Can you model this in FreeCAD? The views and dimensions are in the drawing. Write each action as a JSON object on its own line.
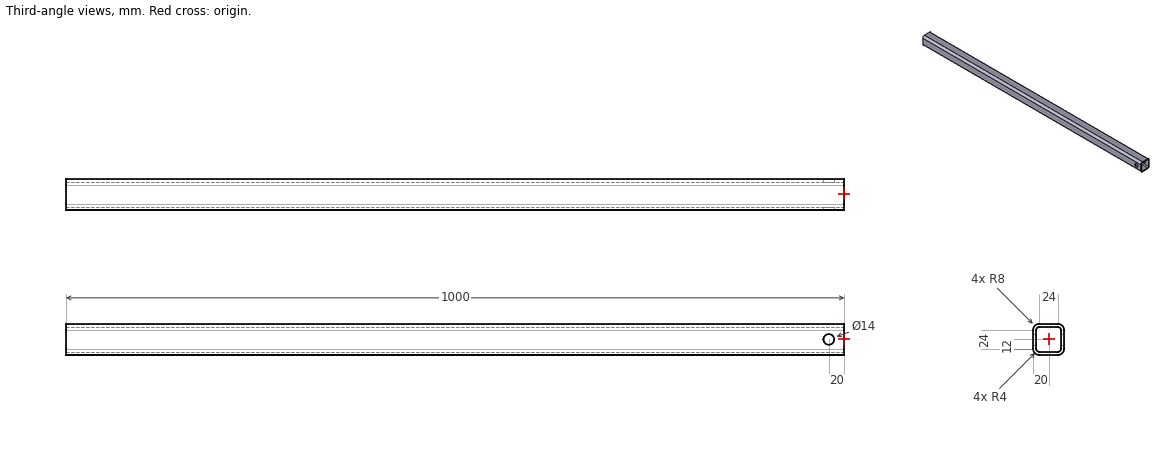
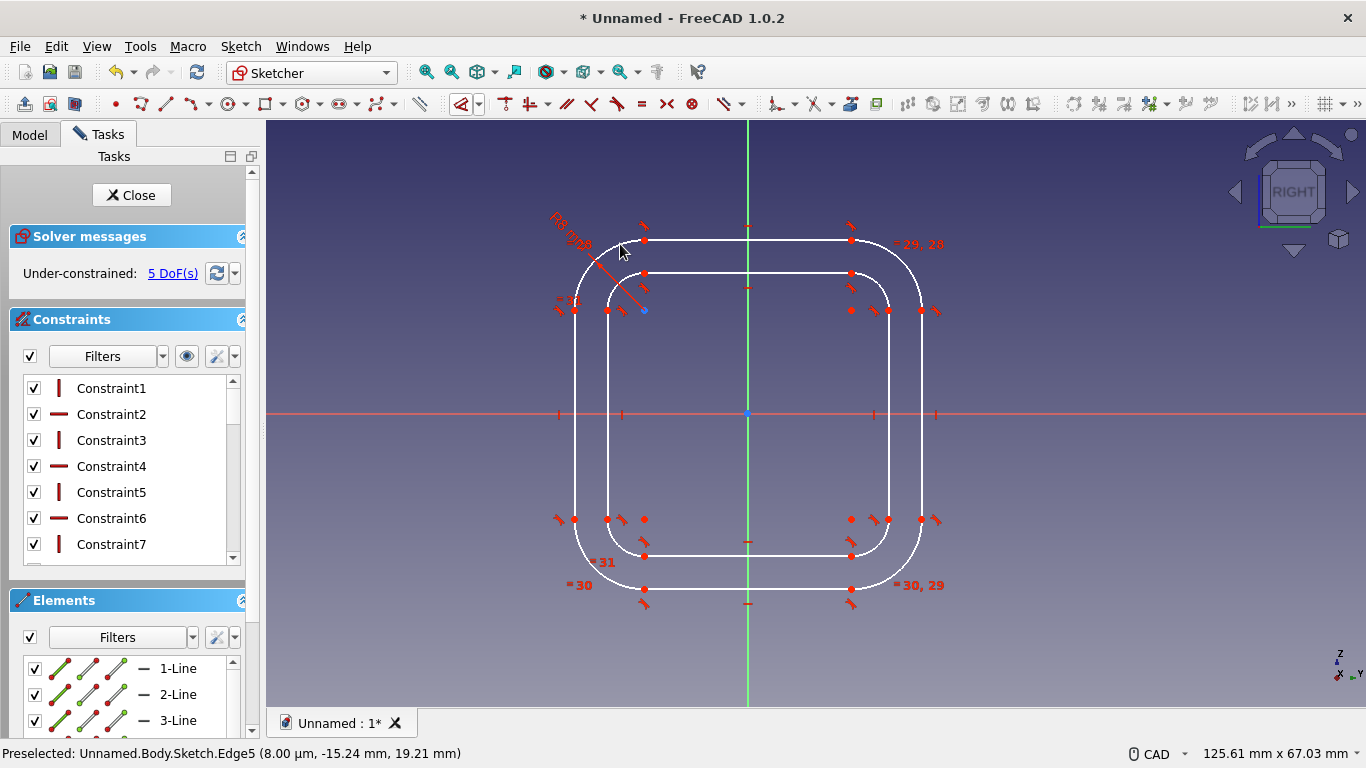
{"action": "left_click", "coordinate": [612, 536]}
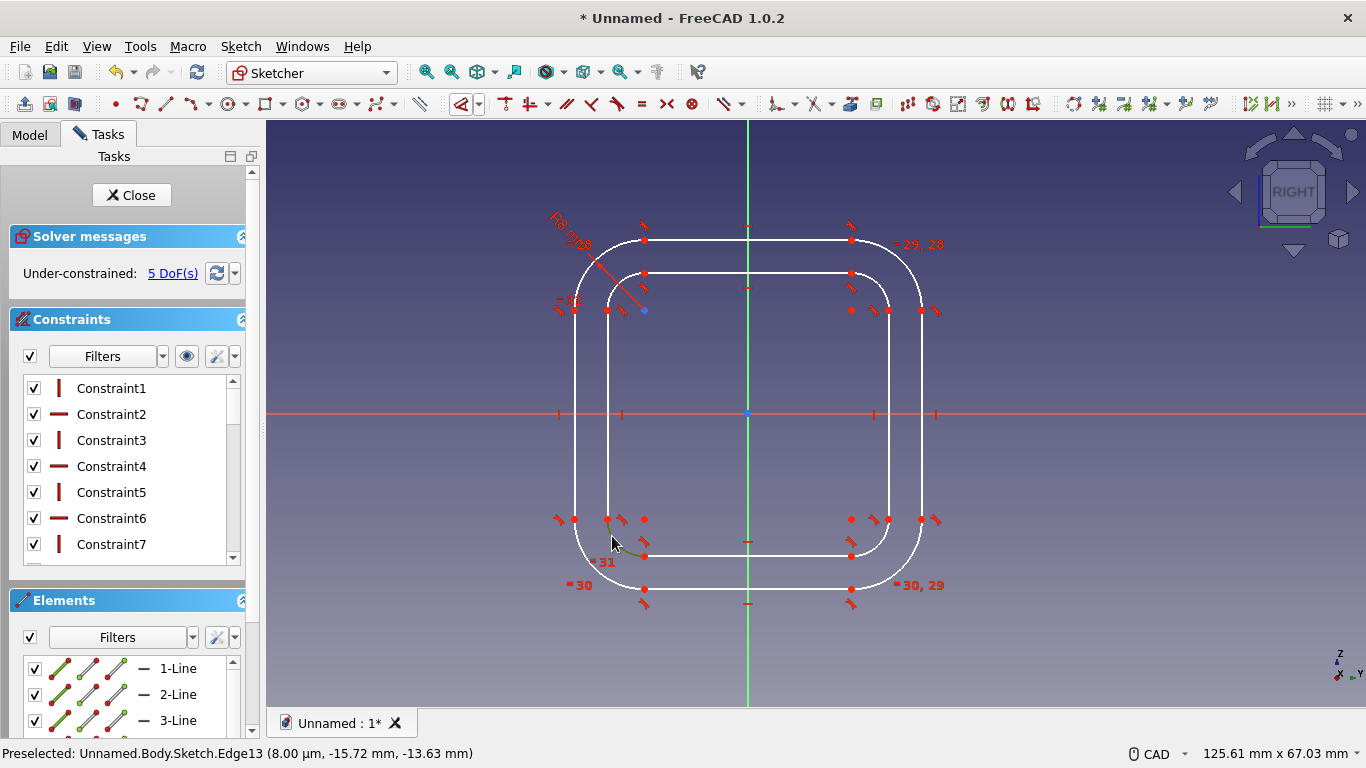
{"action": "left_click", "coordinate": [478, 104]}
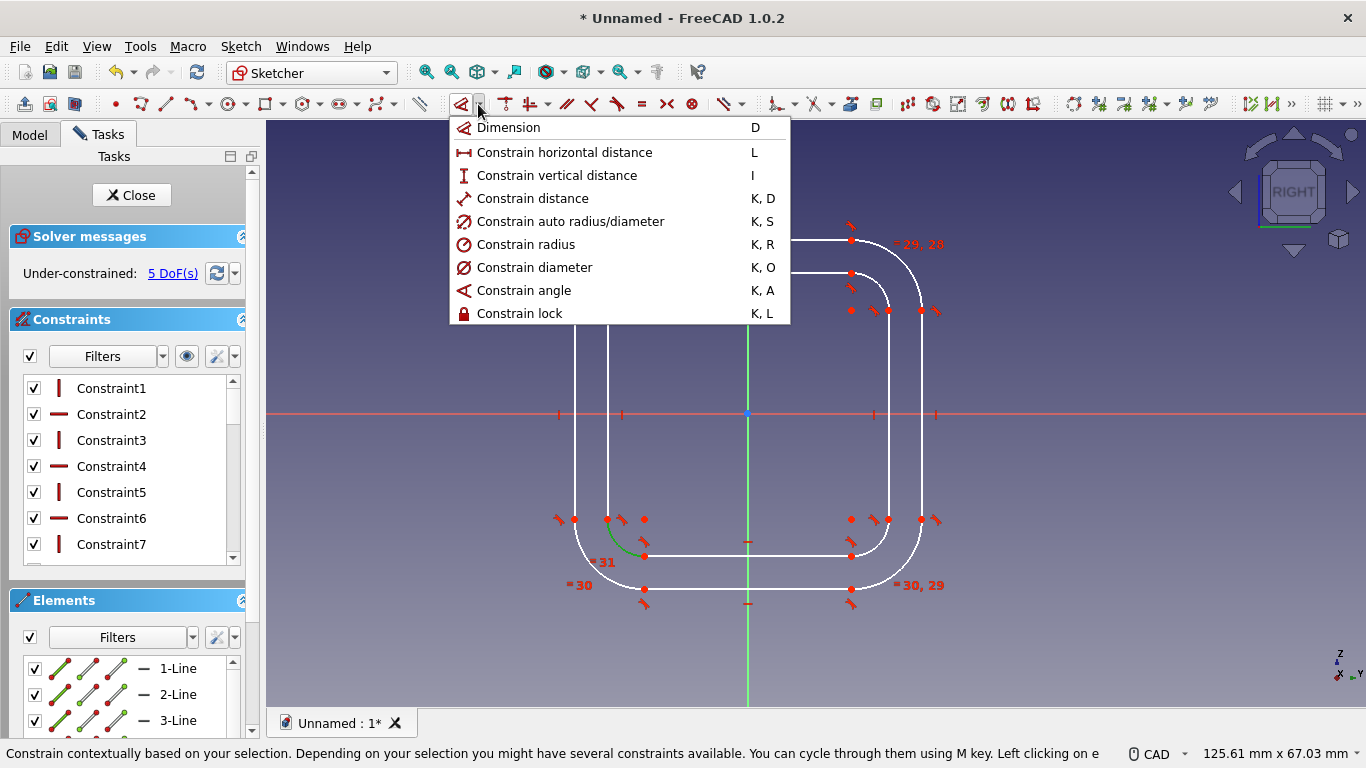
{"action": "left_click", "coordinate": [620, 244]}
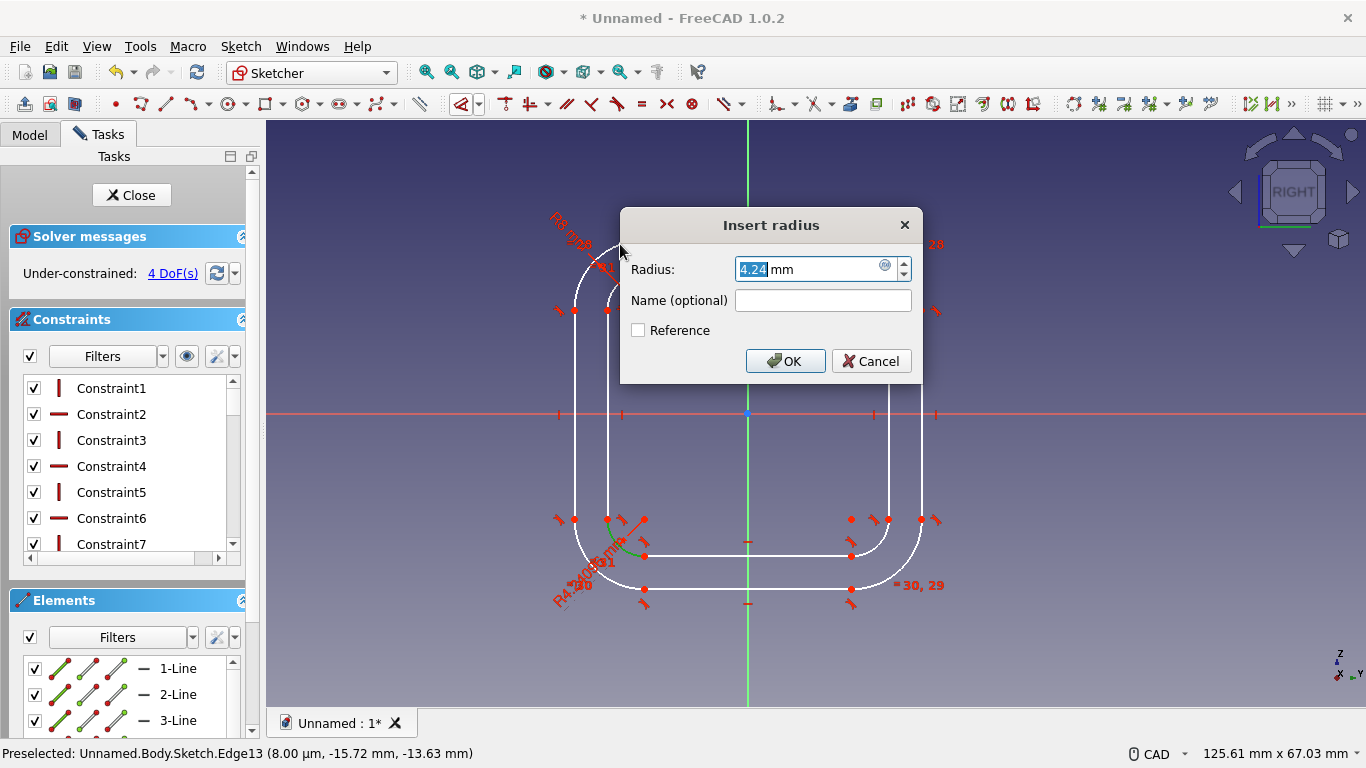
{"action": "type", "text": "4"}
{"action": "key", "text": "Return"}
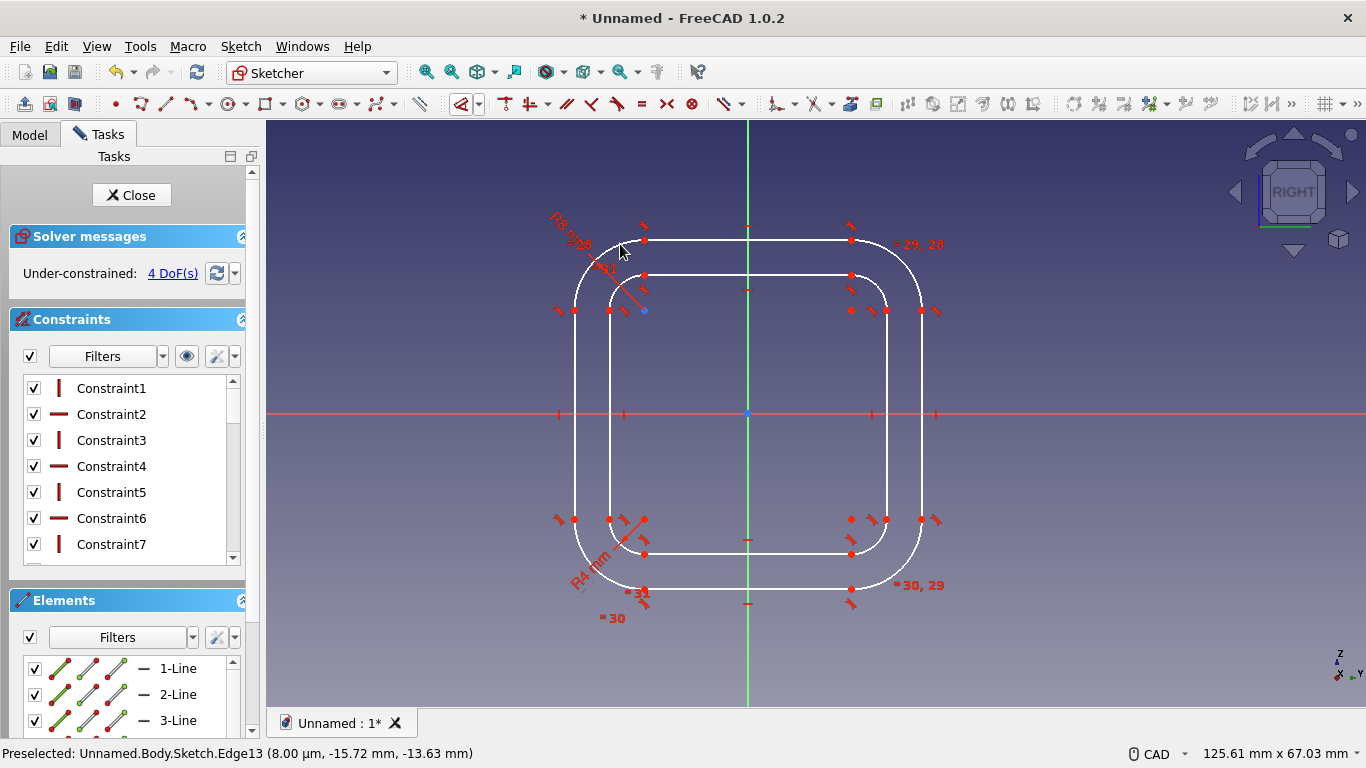
{"action": "left_click", "coordinate": [575, 456]}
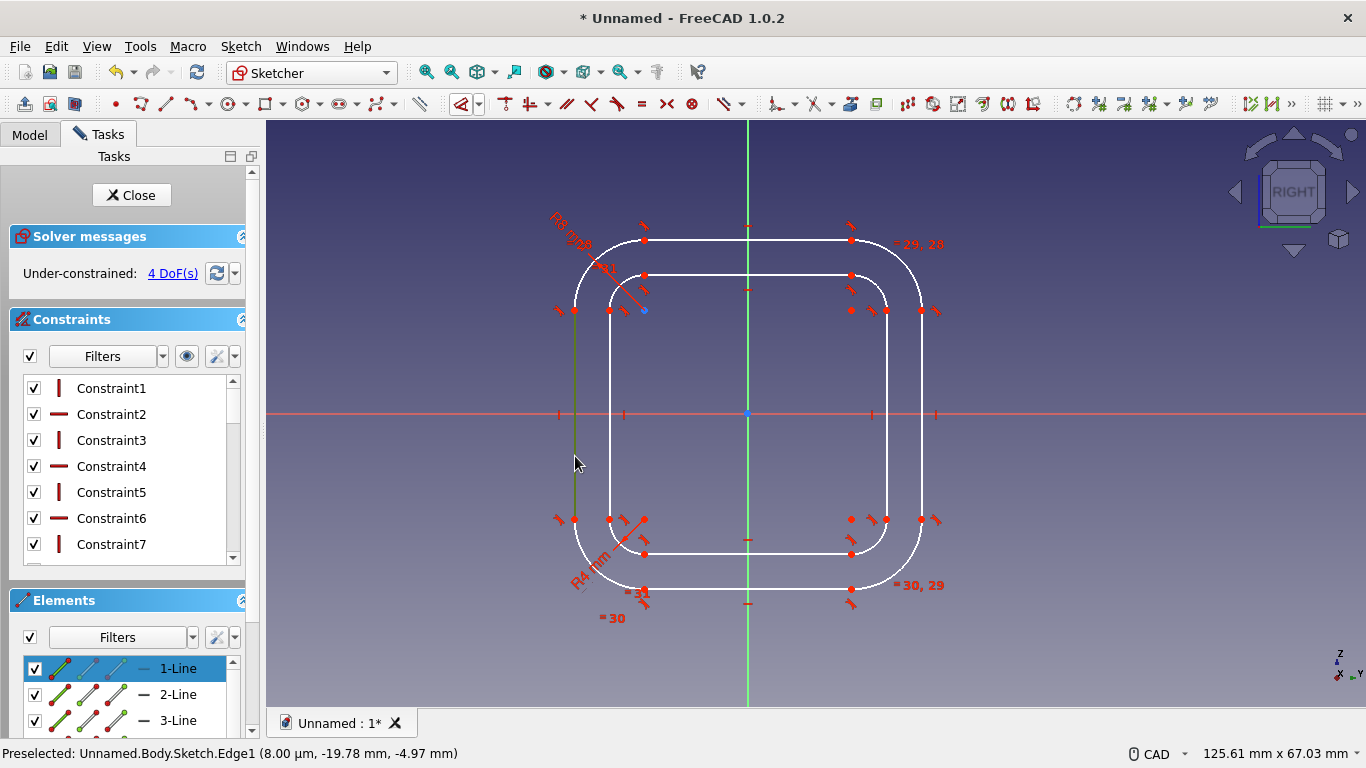
{"action": "left_click", "coordinate": [478, 104]}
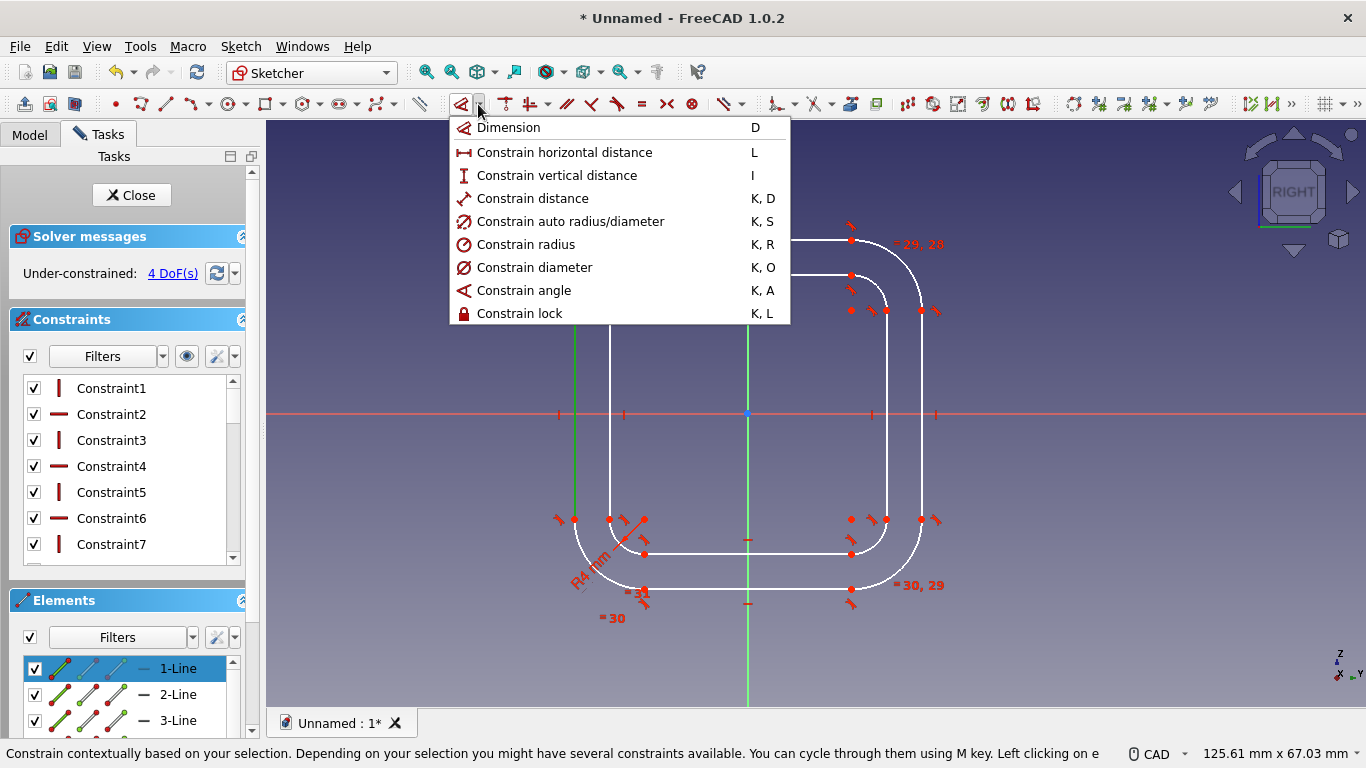
{"action": "left_click", "coordinate": [620, 176]}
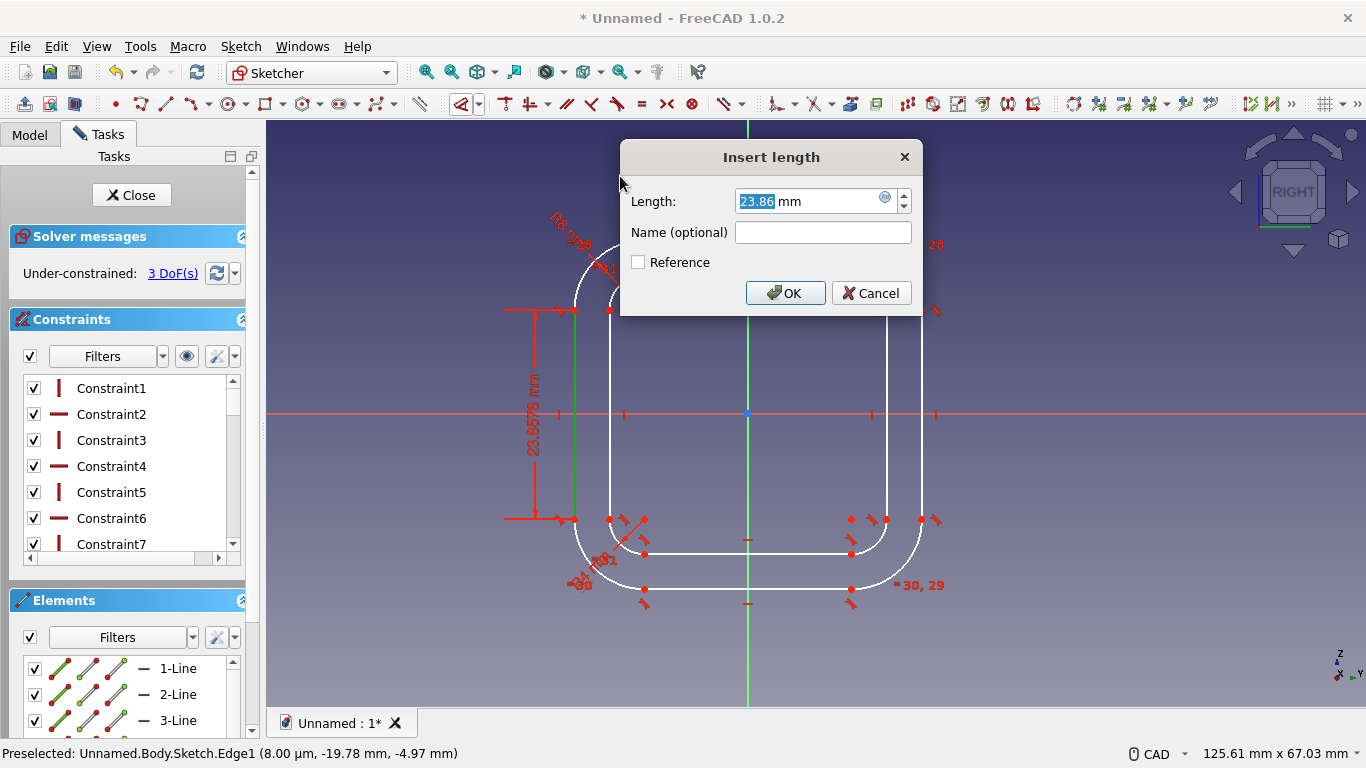
{"action": "type", "text": "24"}
{"action": "key", "text": "Return"}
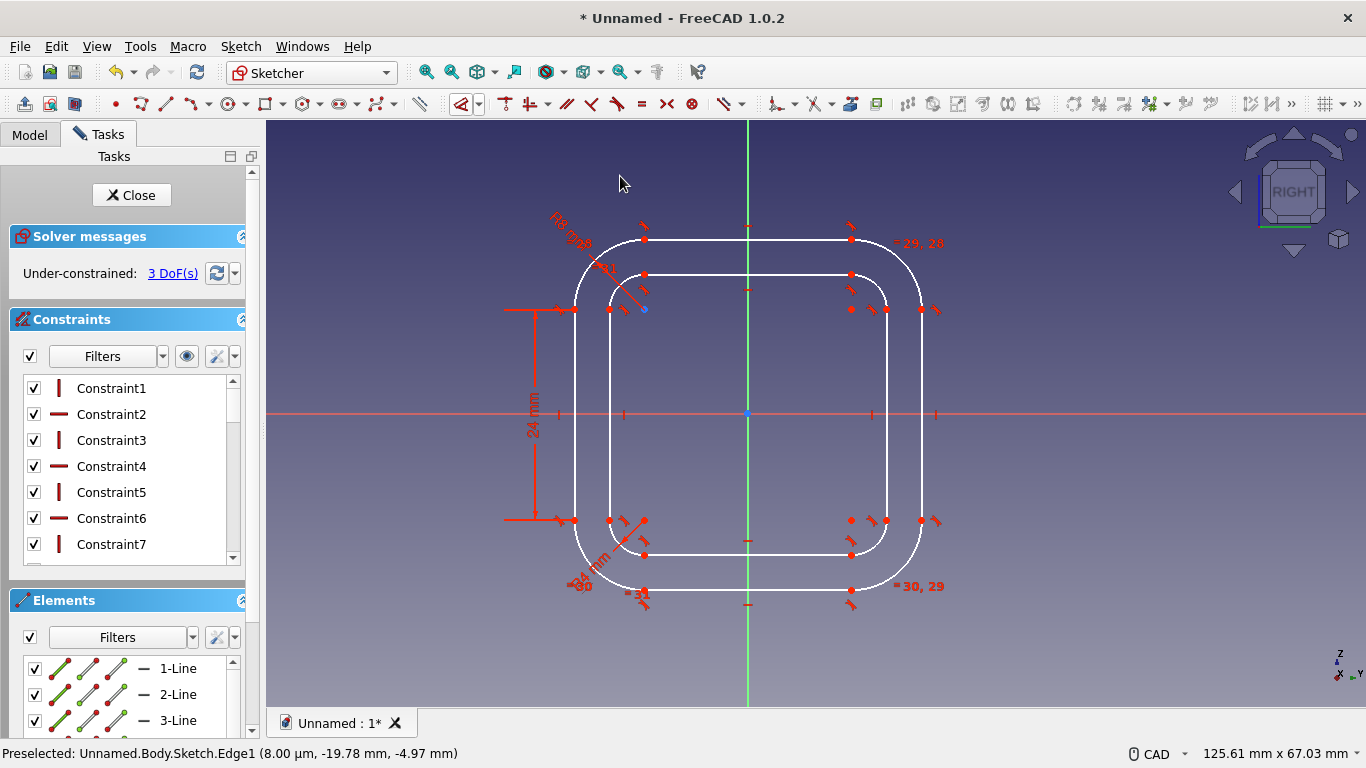
{"action": "left_click", "coordinate": [707, 240]}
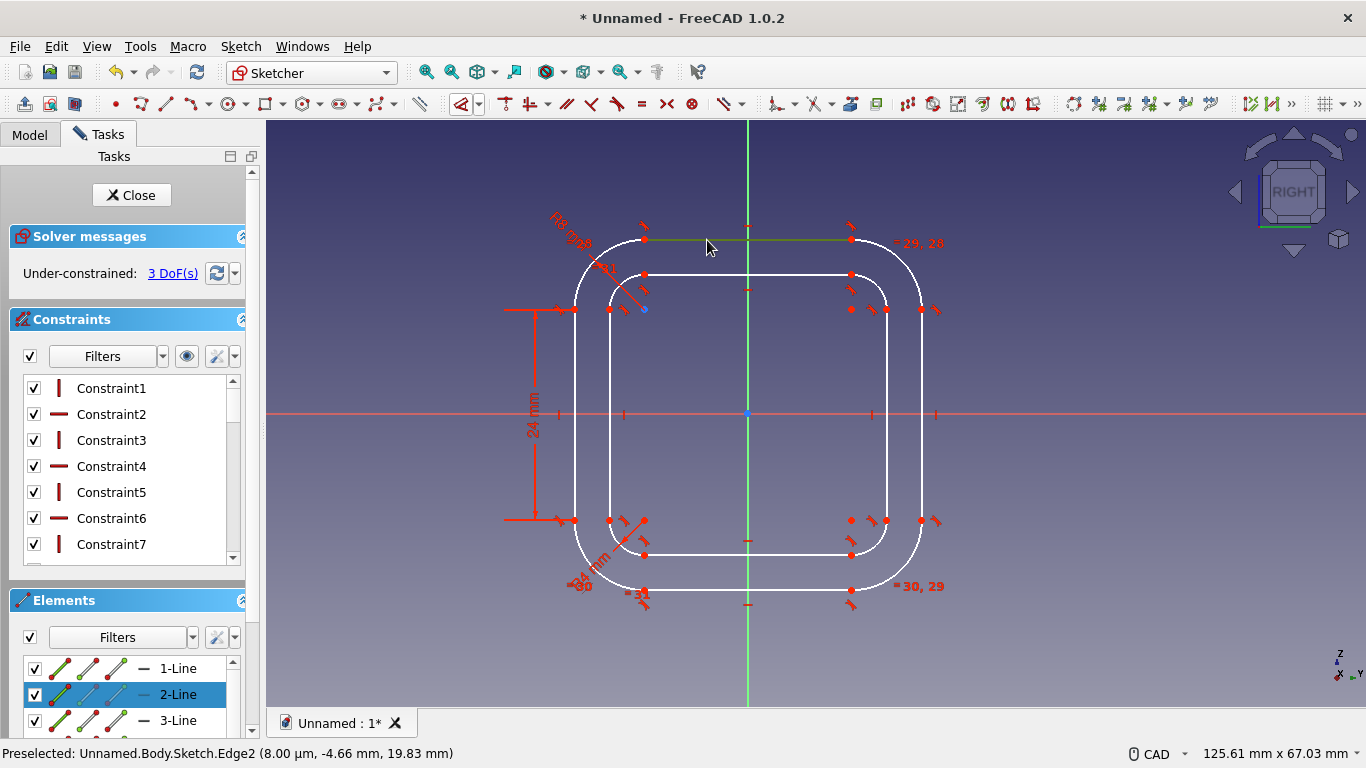
{"action": "key", "text": "l"}